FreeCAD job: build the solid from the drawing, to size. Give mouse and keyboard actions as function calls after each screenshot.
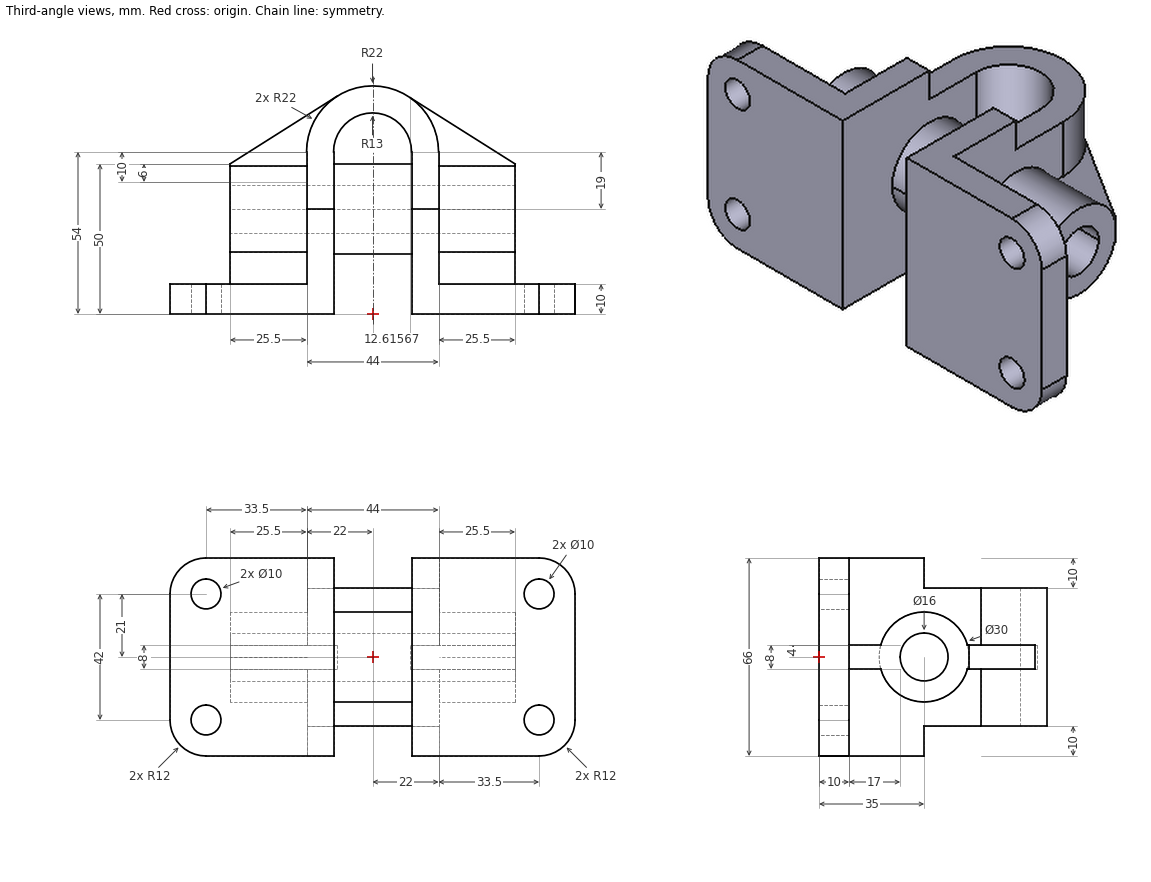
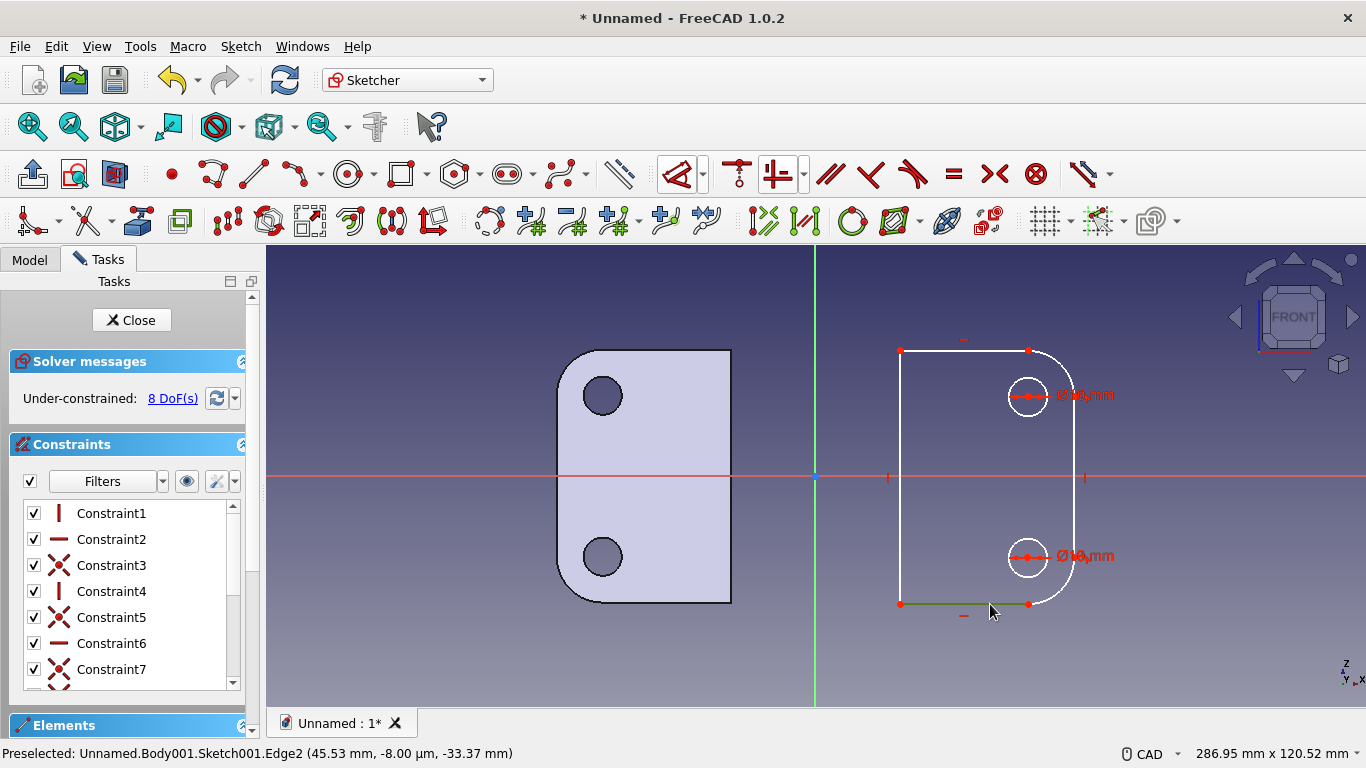
click(1049, 599)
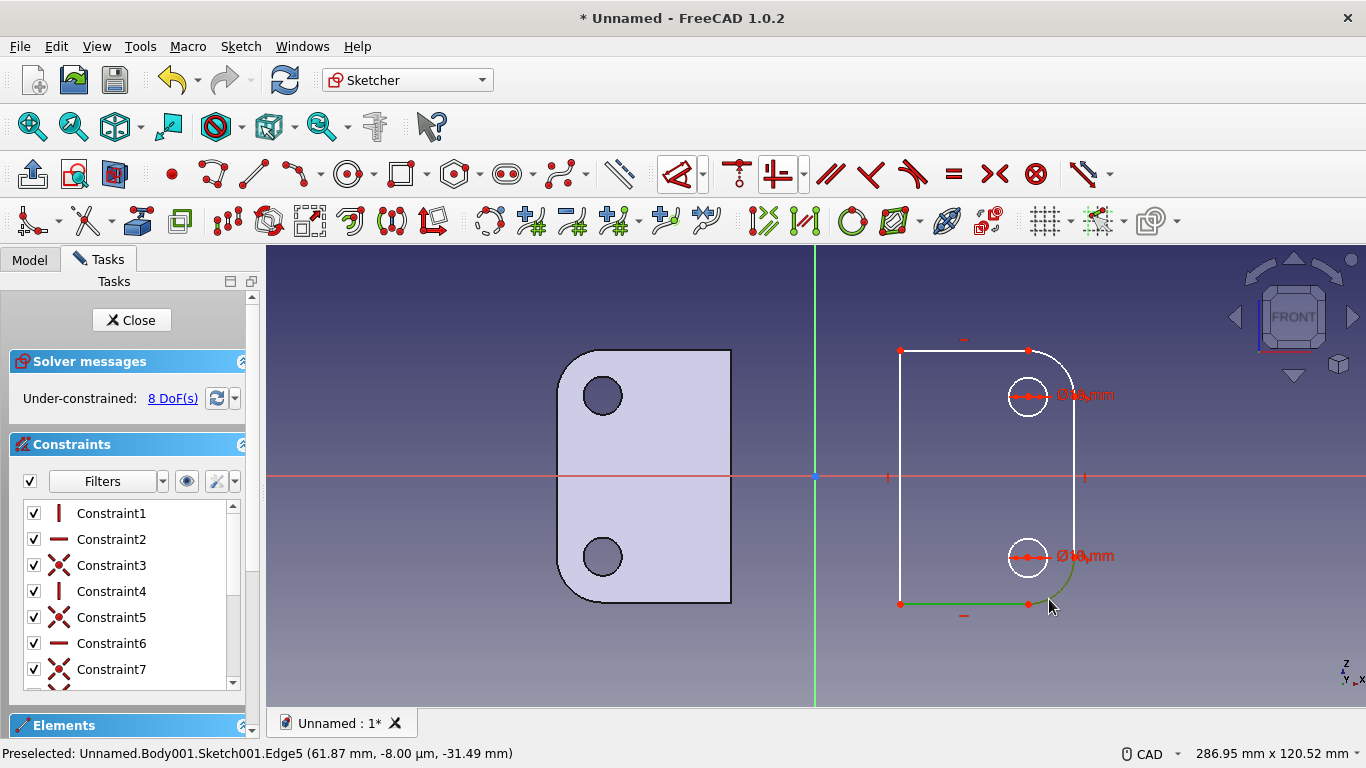
click(913, 174)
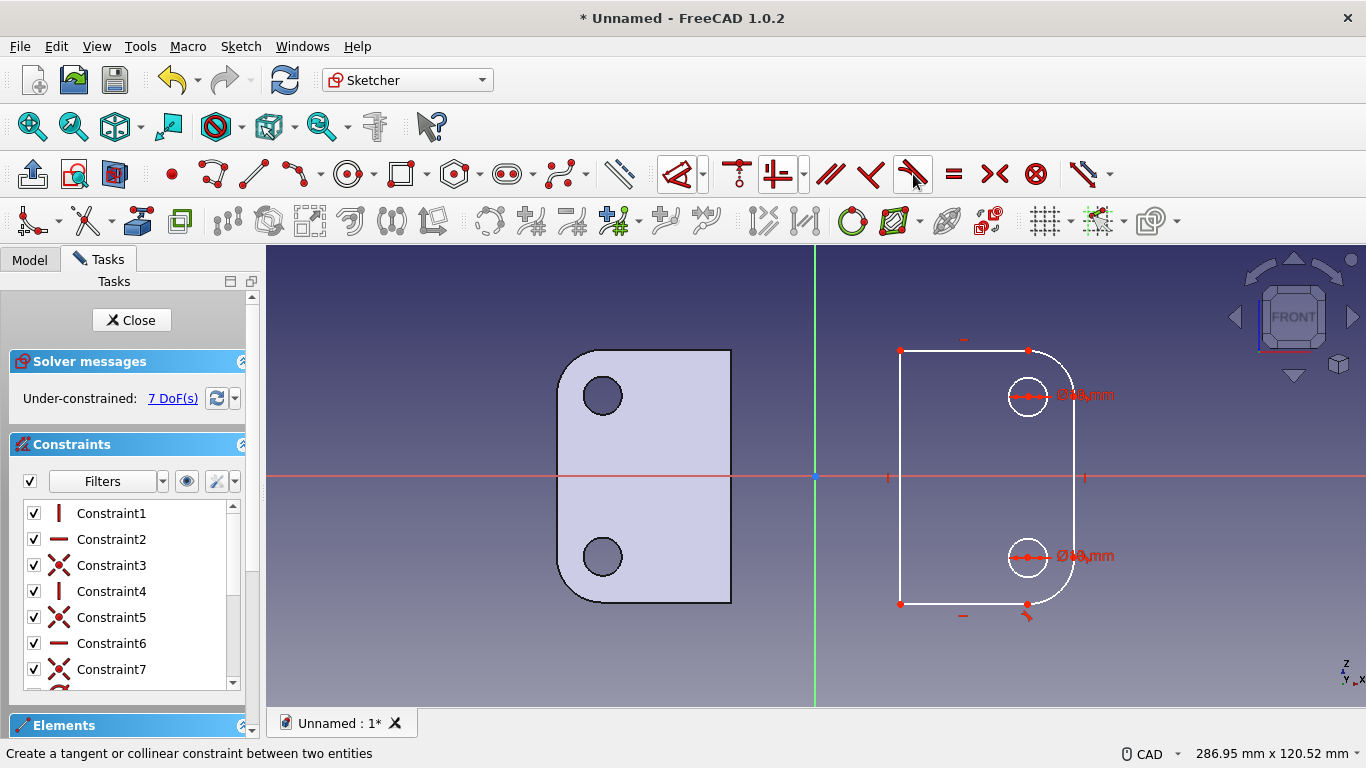
click(938, 351)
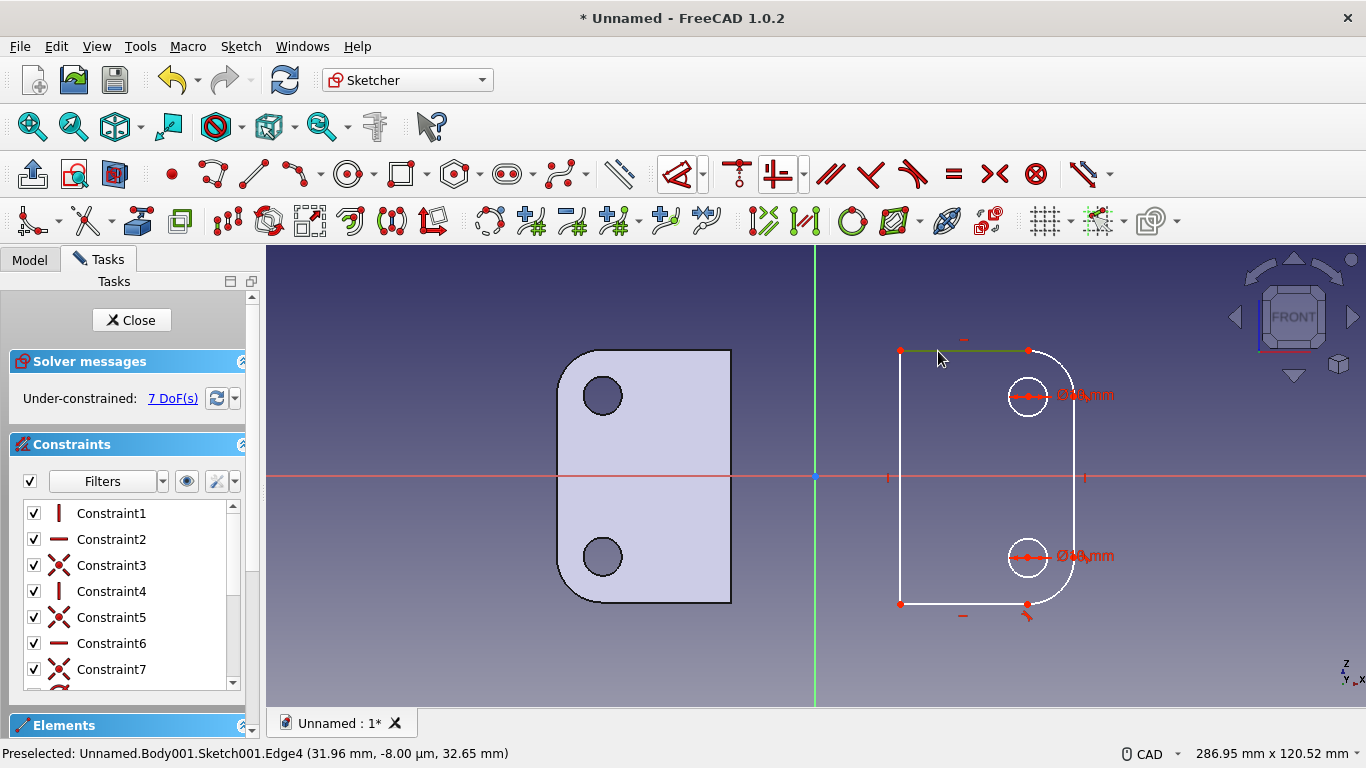
click(1069, 376)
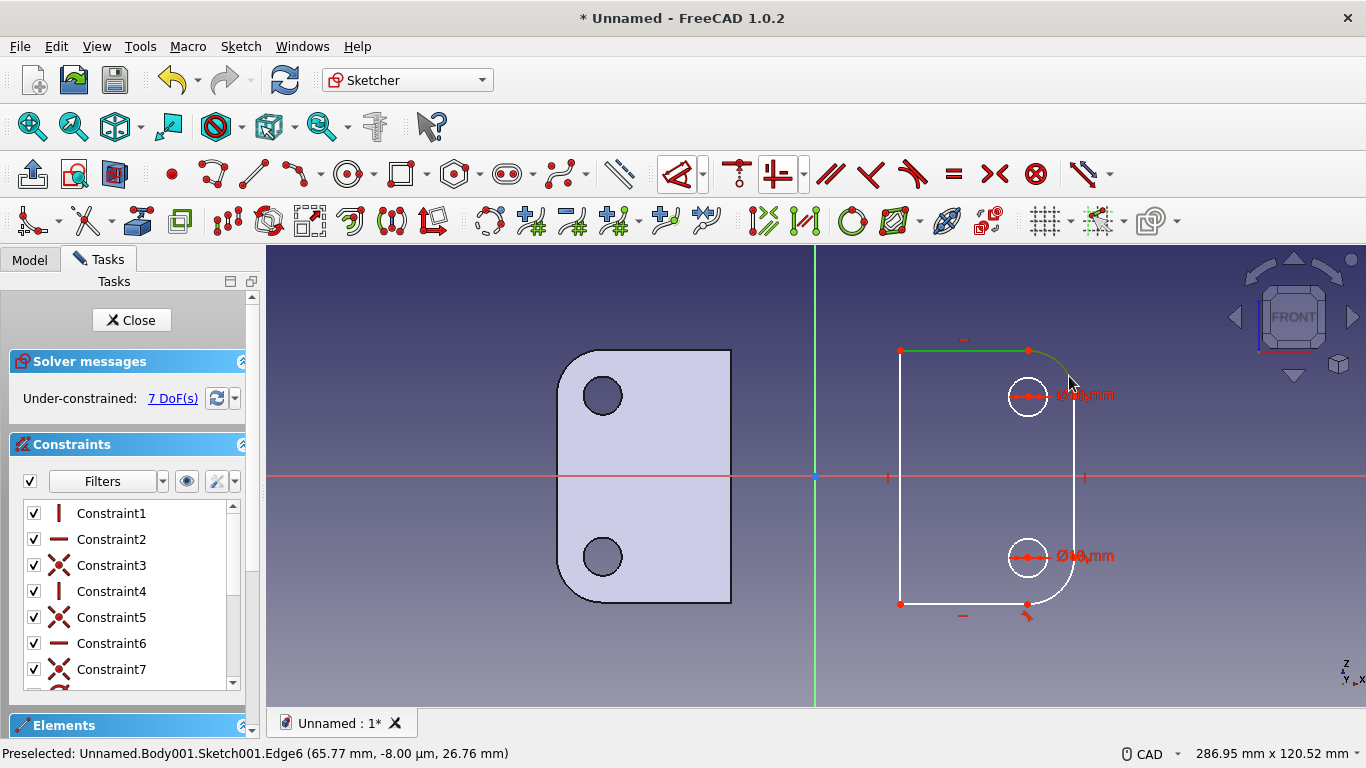
click(913, 174)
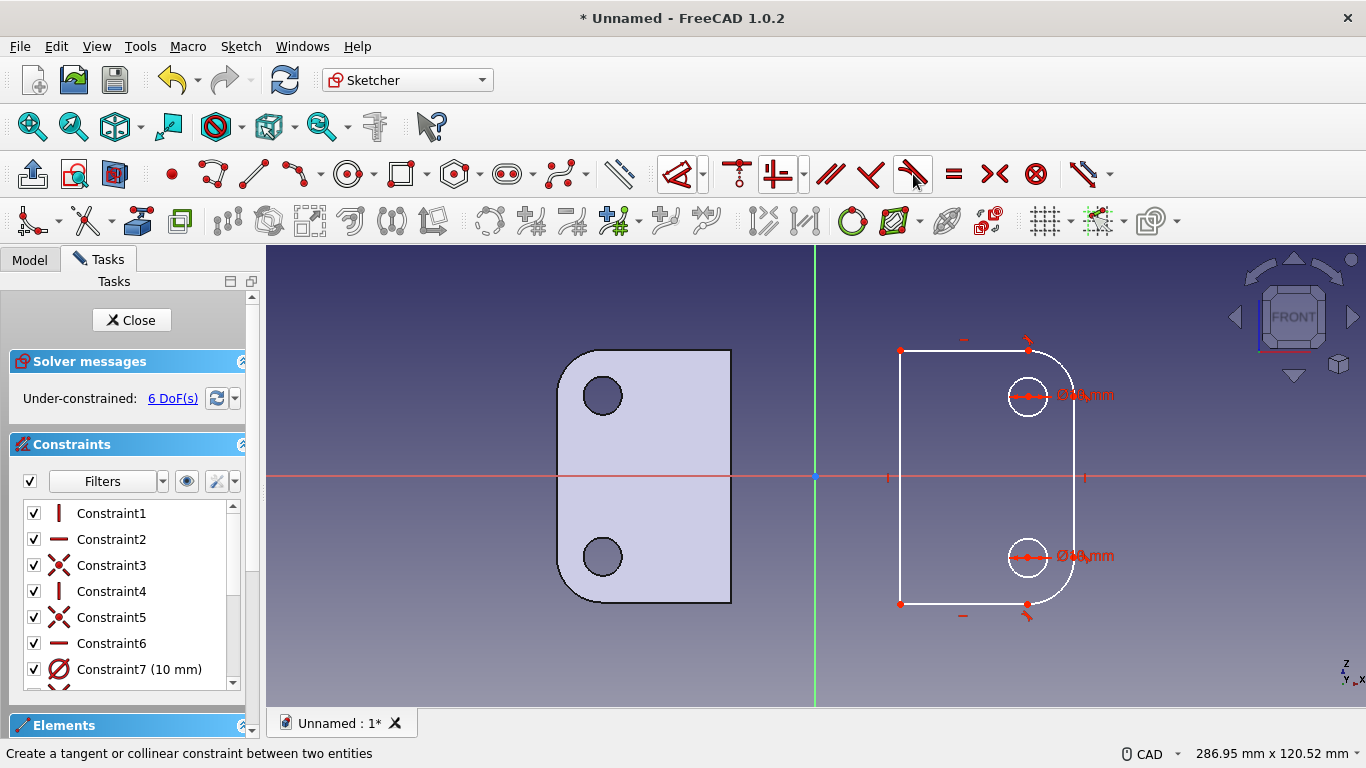
click(1049, 599)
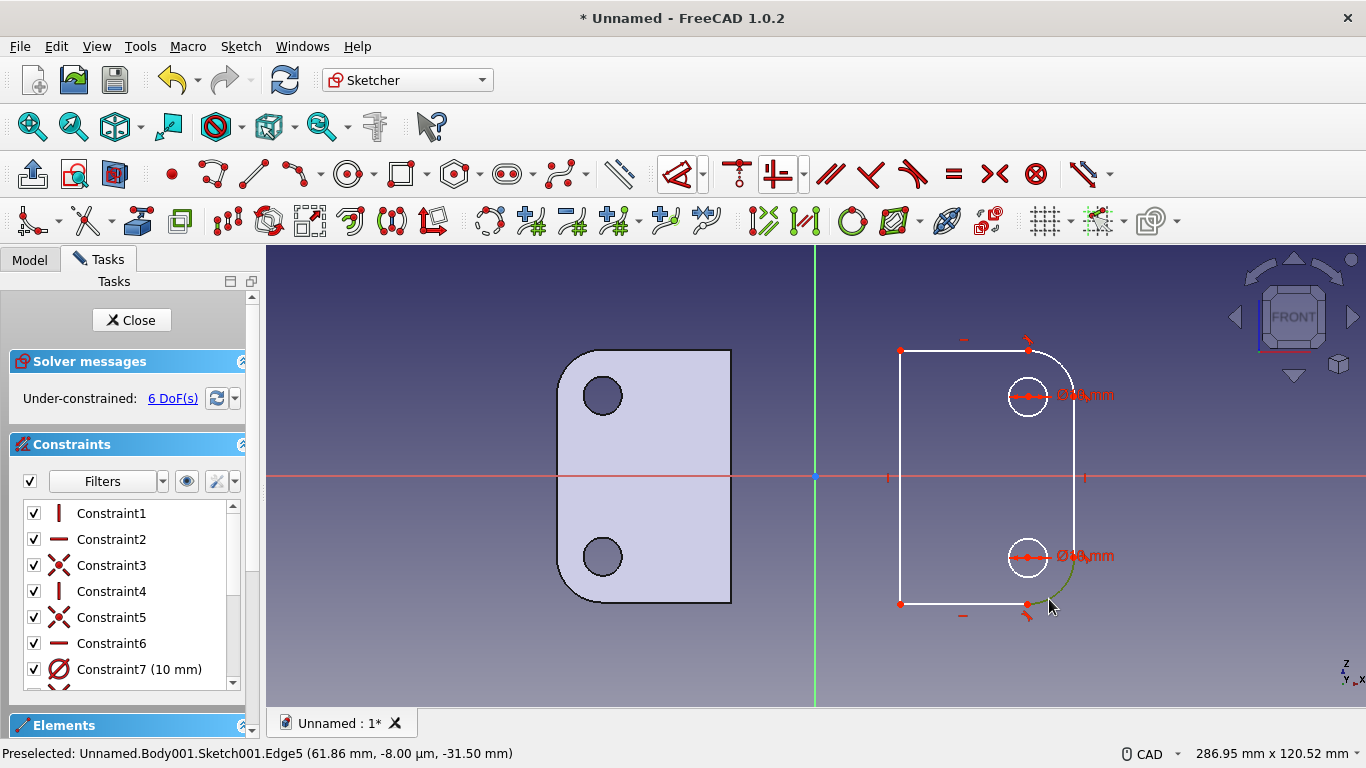
click(1069, 376)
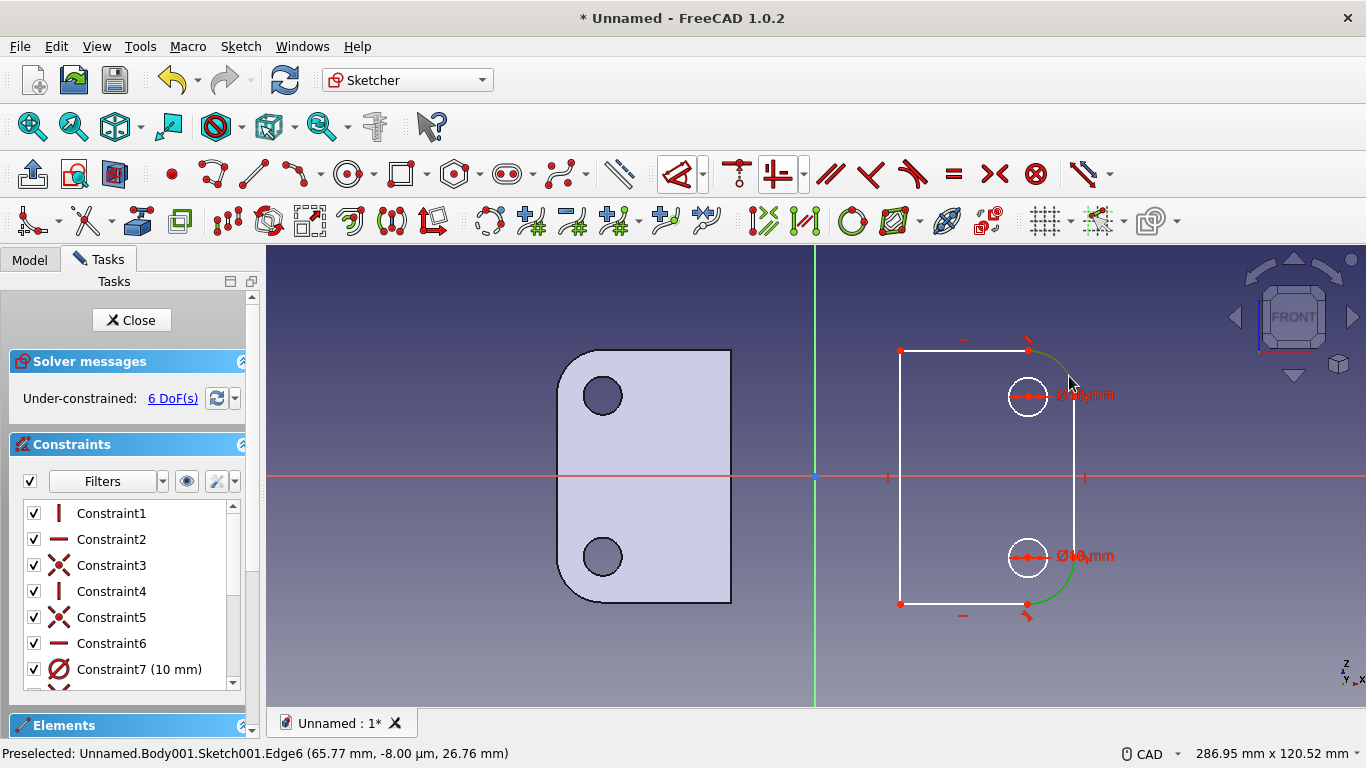
click(954, 174)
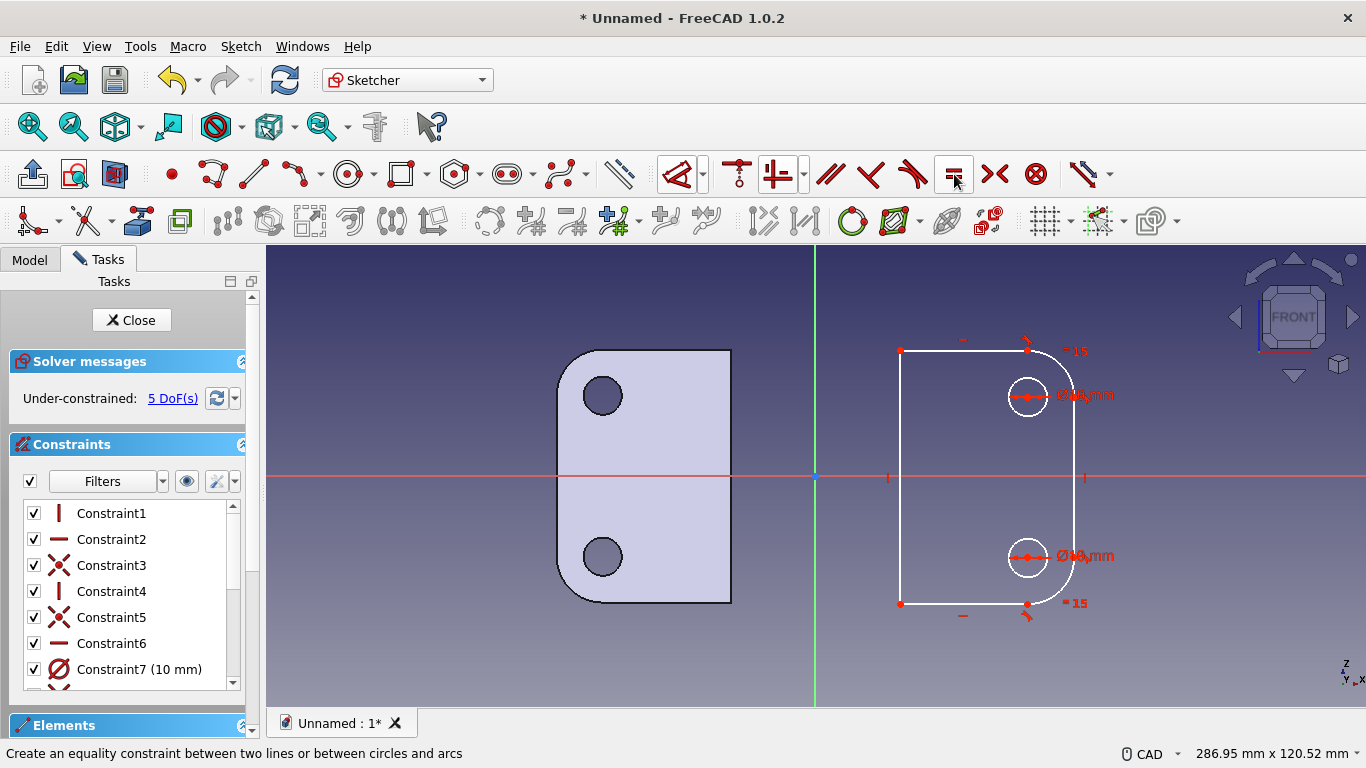
click(1049, 599)